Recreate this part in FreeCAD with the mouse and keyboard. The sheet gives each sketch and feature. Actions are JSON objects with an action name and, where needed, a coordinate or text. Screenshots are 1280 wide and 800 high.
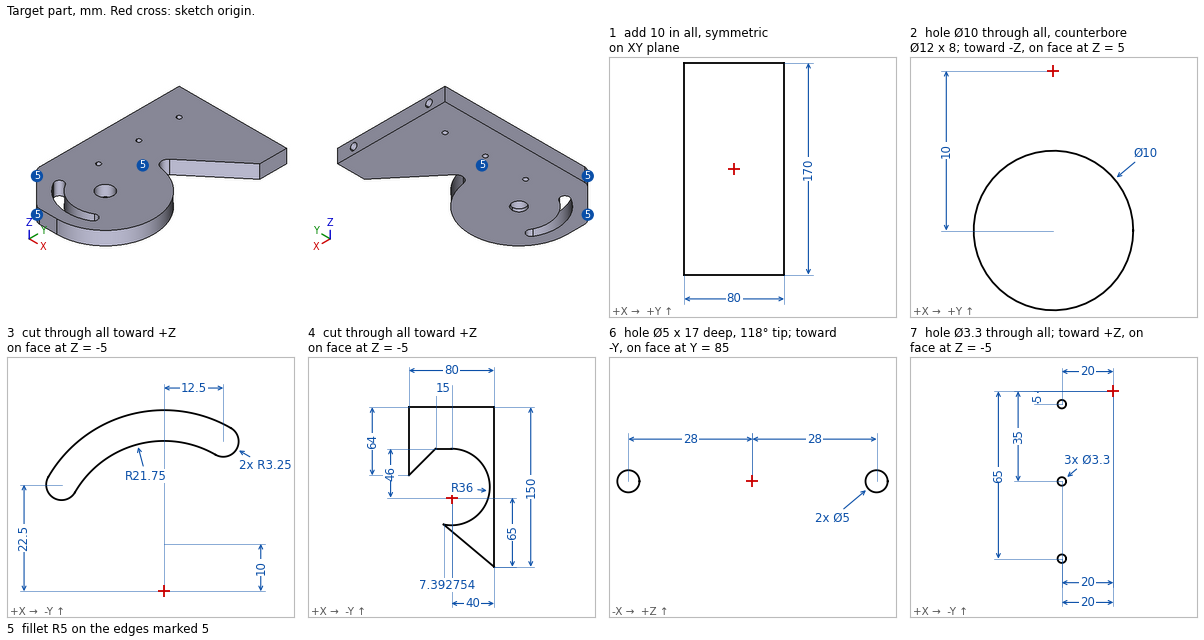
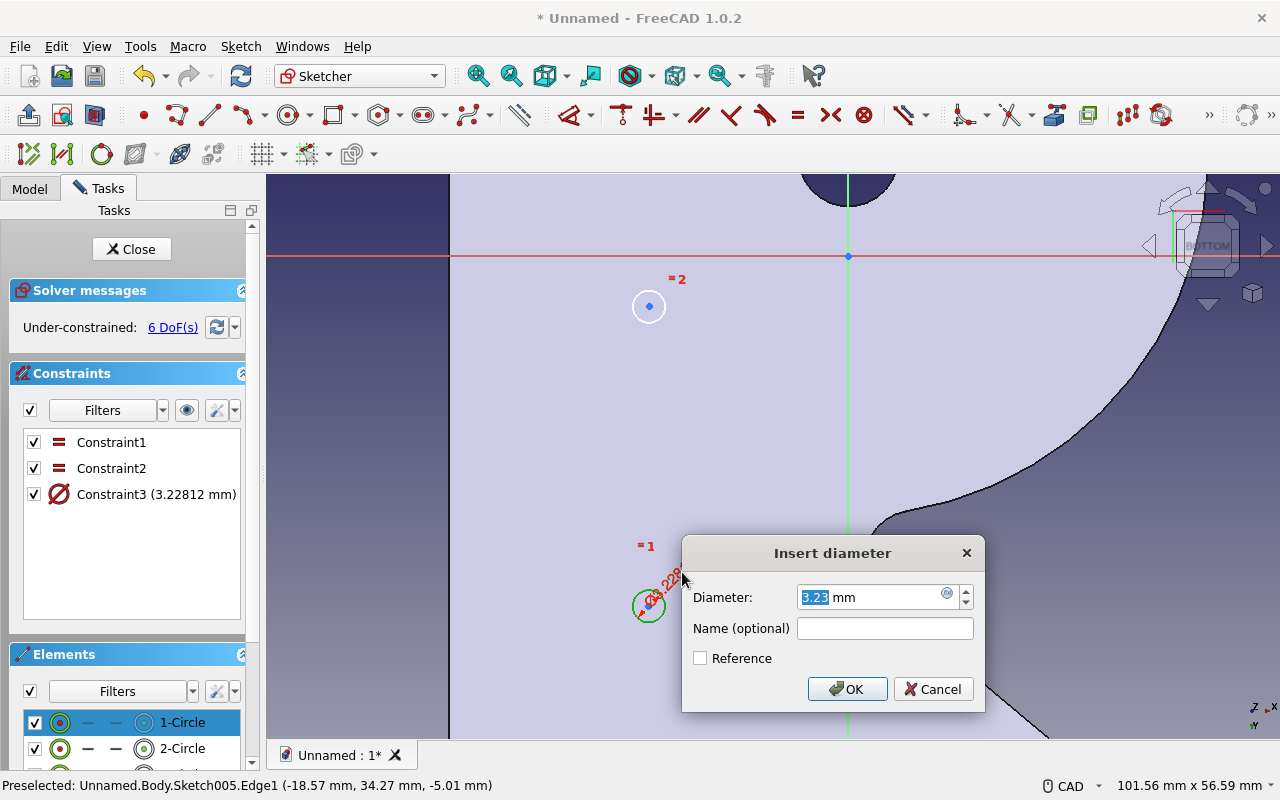
{"action": "type", "text": "3.3"}
{"action": "key", "text": "Return"}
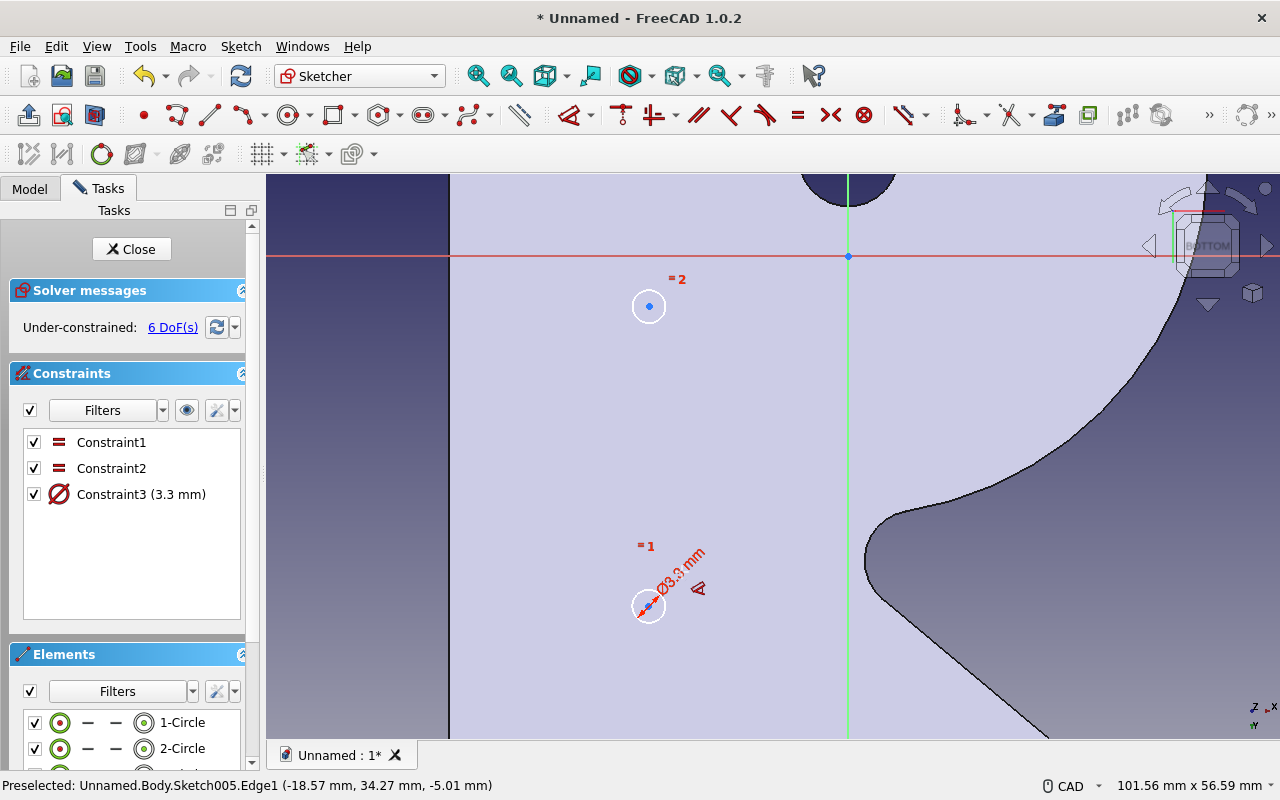
{"action": "left_click", "coordinate": [649, 307]}
{"action": "left_click", "coordinate": [882, 282]}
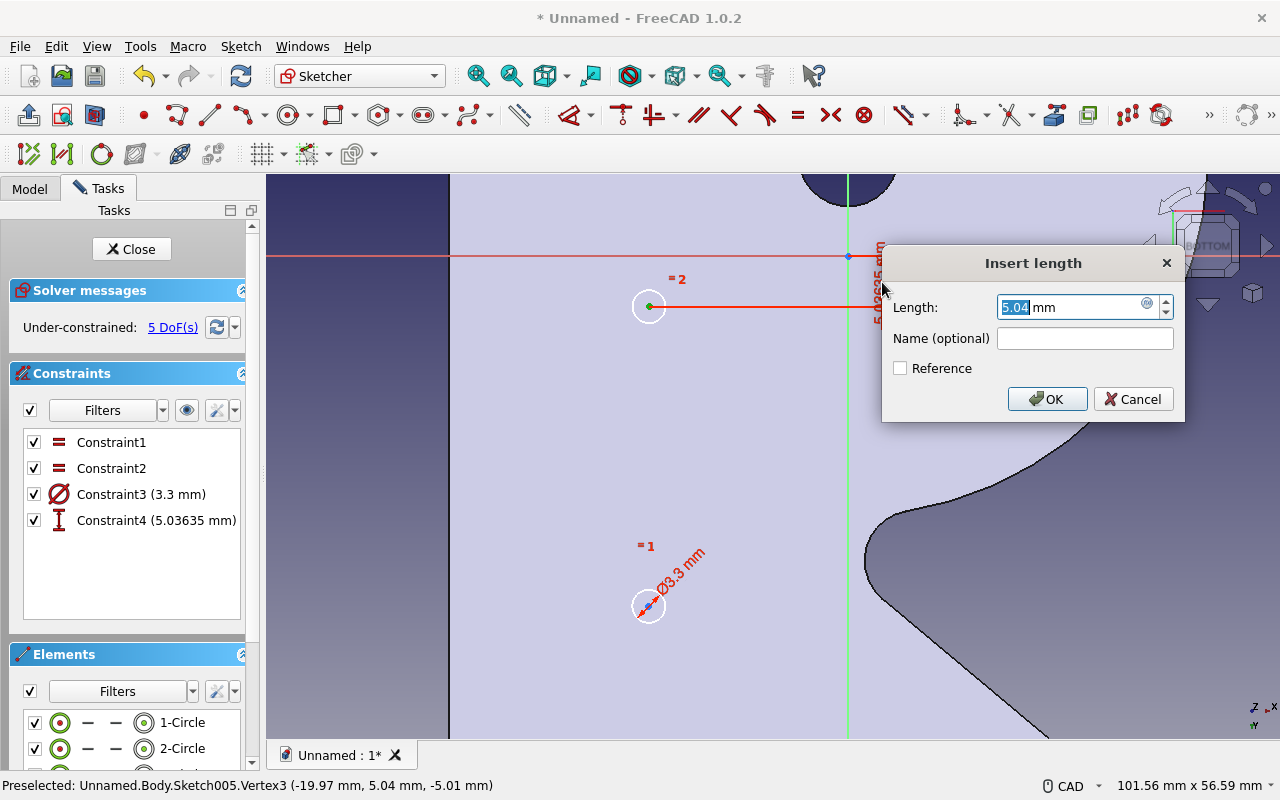
{"action": "type", "text": "5"}
{"action": "key", "text": "Return"}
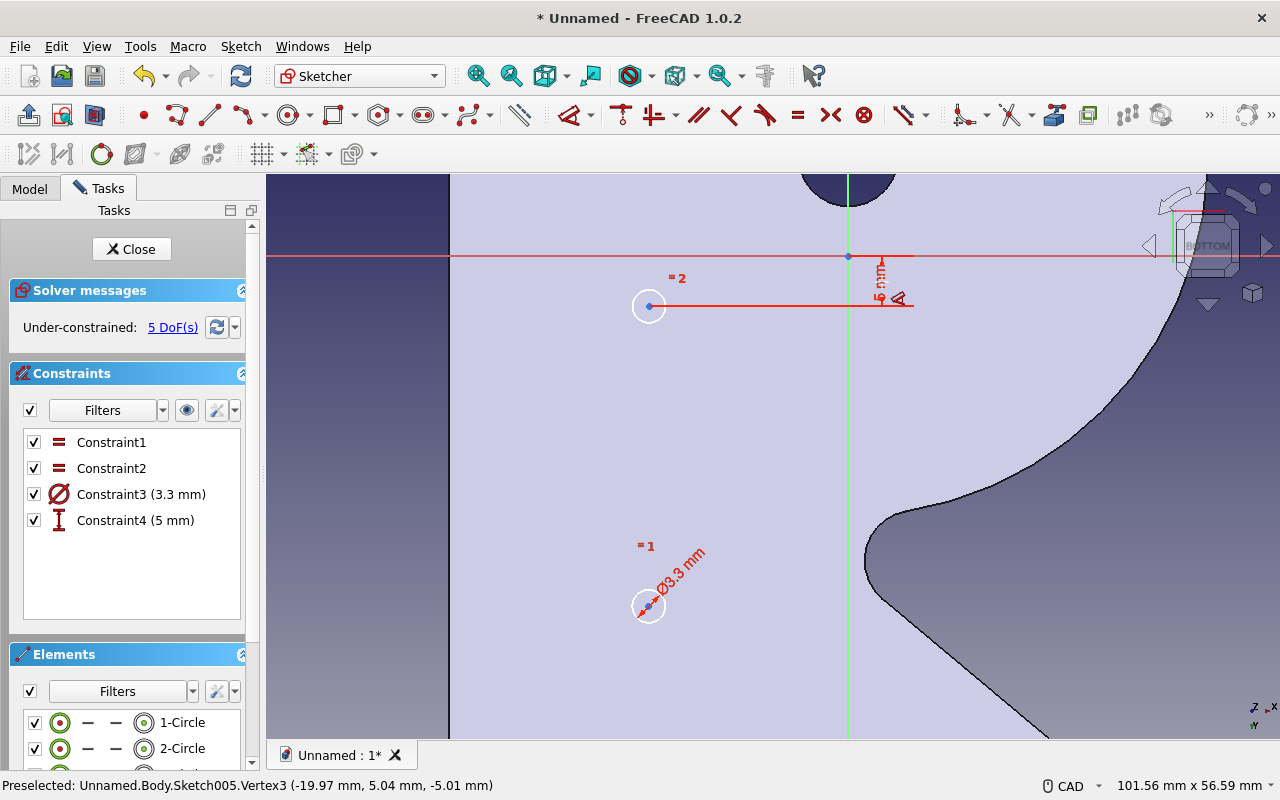
{"action": "left_click", "coordinate": [649, 606]}
{"action": "left_click", "coordinate": [749, 222]}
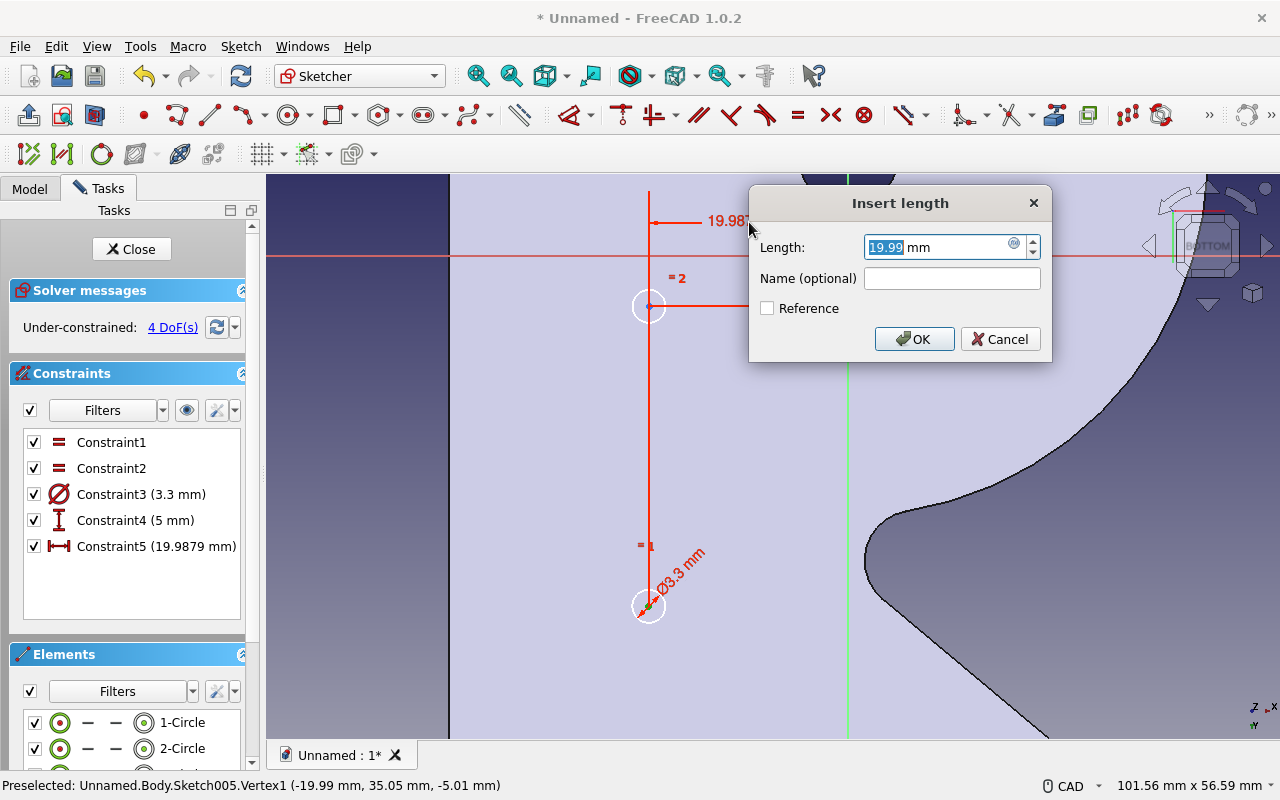
{"action": "type", "text": "20"}
{"action": "key", "text": "Return"}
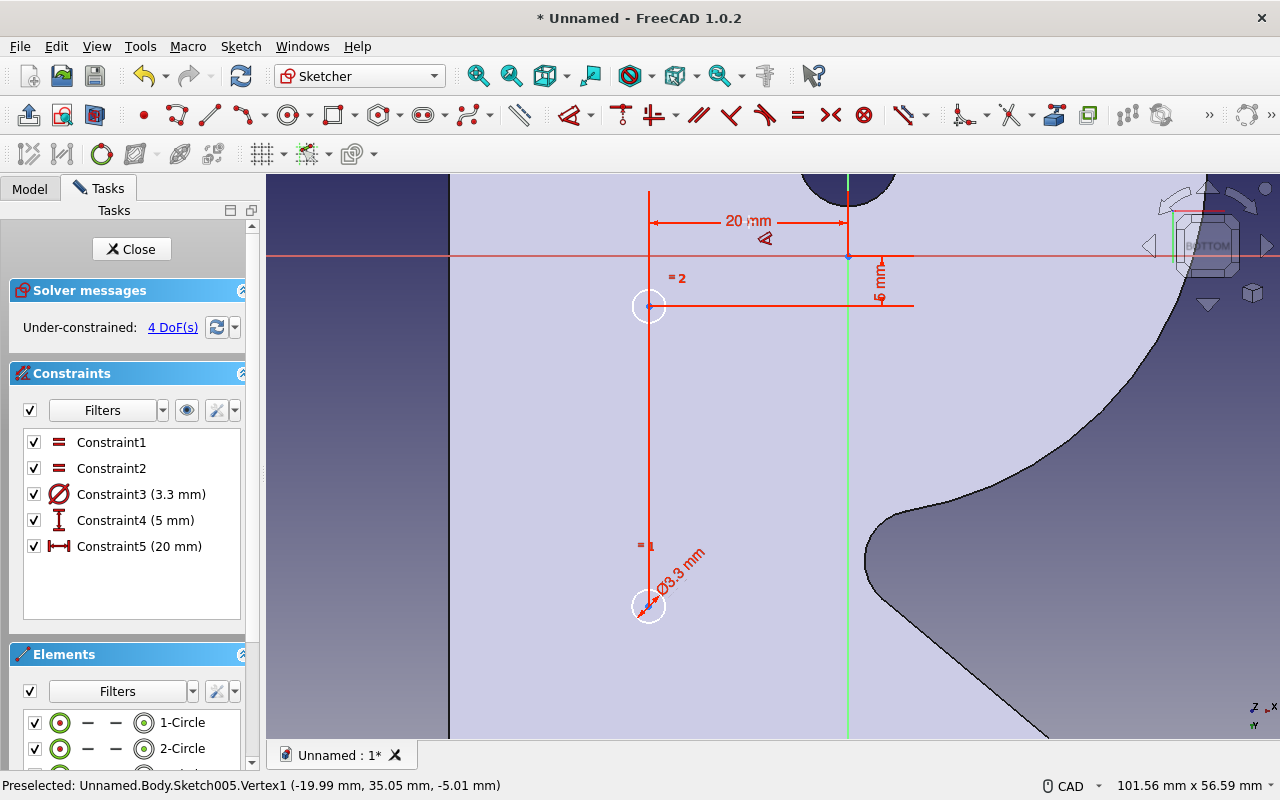
{"action": "left_click", "coordinate": [649, 606]}
{"action": "left_click", "coordinate": [882, 431]}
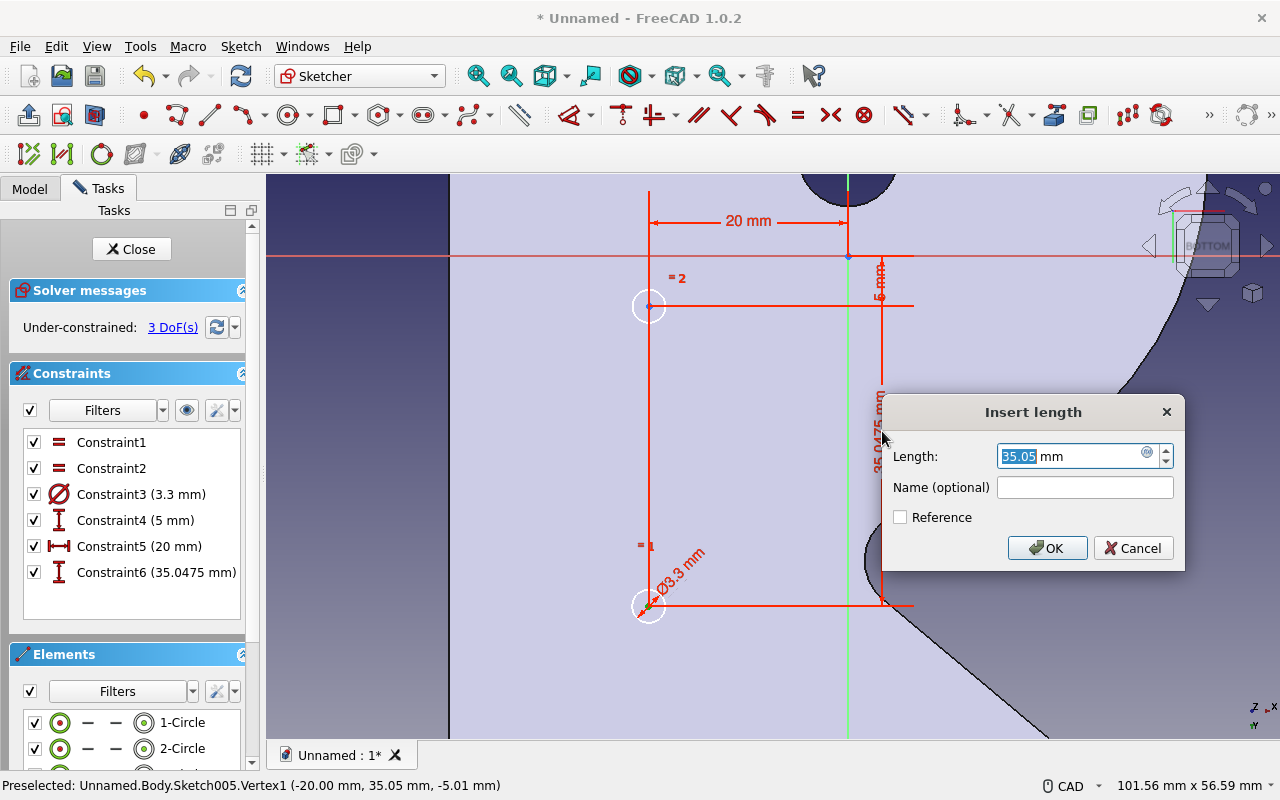
{"action": "type", "text": "35"}
{"action": "key", "text": "Return"}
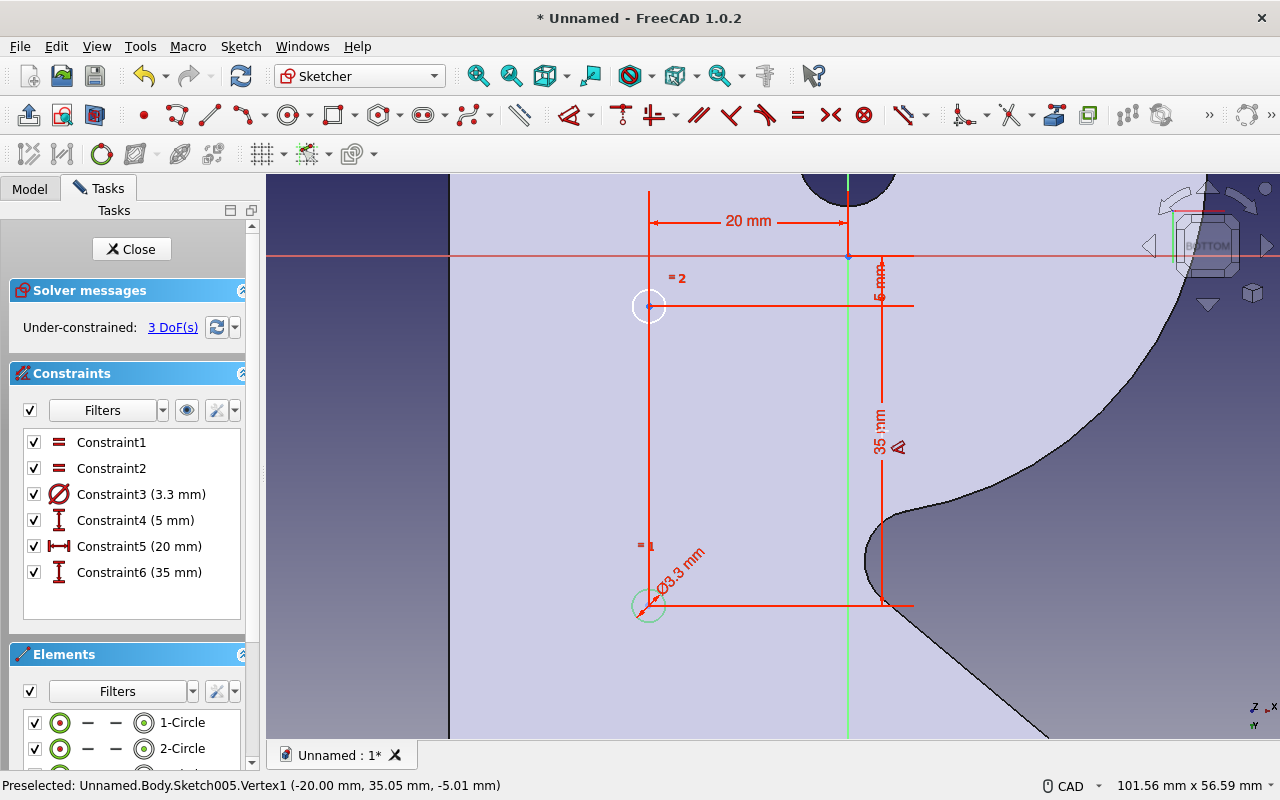
{"action": "scroll", "coordinate": [661, 295], "scroll_direction": "down", "scroll_amount": 3}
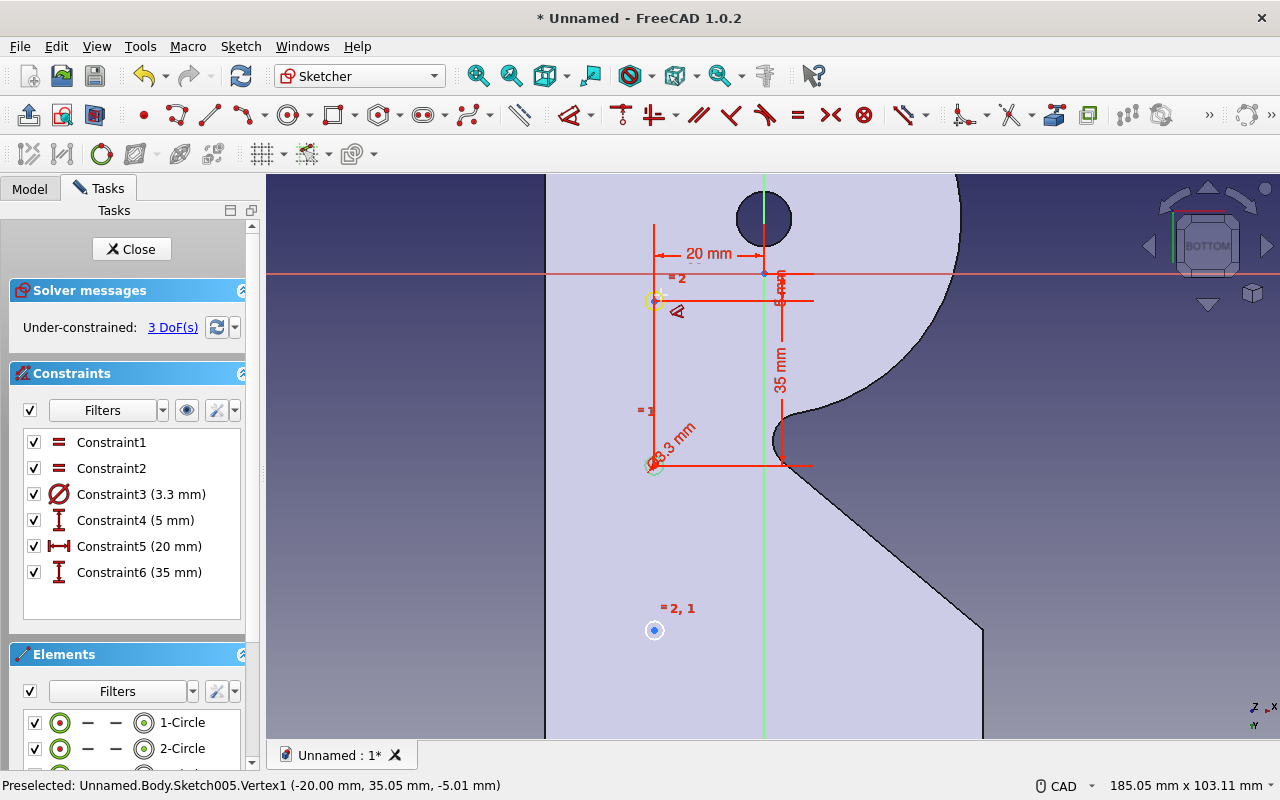
{"action": "left_click", "coordinate": [655, 631]}
{"action": "left_click", "coordinate": [709, 665]}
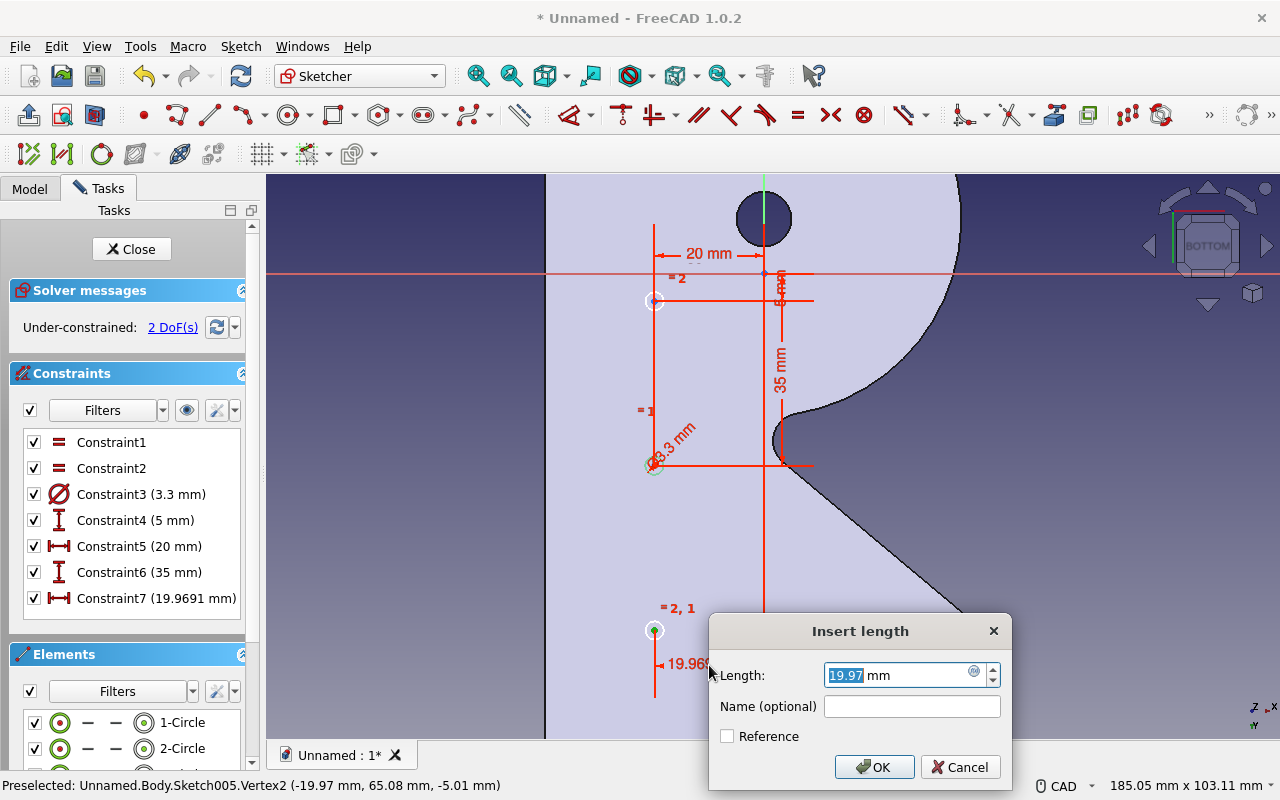
{"action": "type", "text": "20"}
{"action": "key", "text": "Return"}